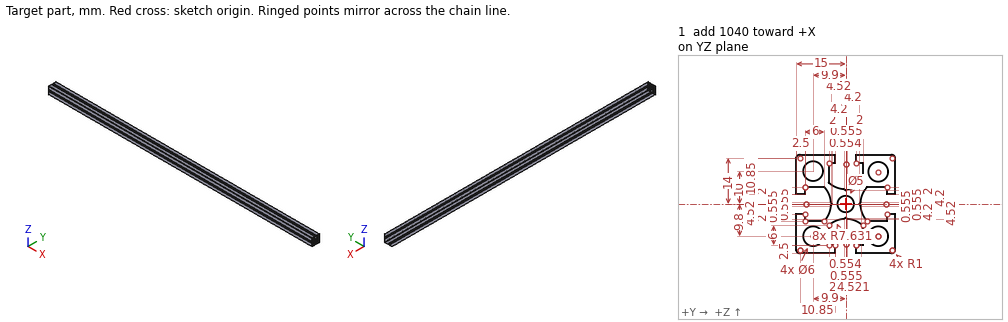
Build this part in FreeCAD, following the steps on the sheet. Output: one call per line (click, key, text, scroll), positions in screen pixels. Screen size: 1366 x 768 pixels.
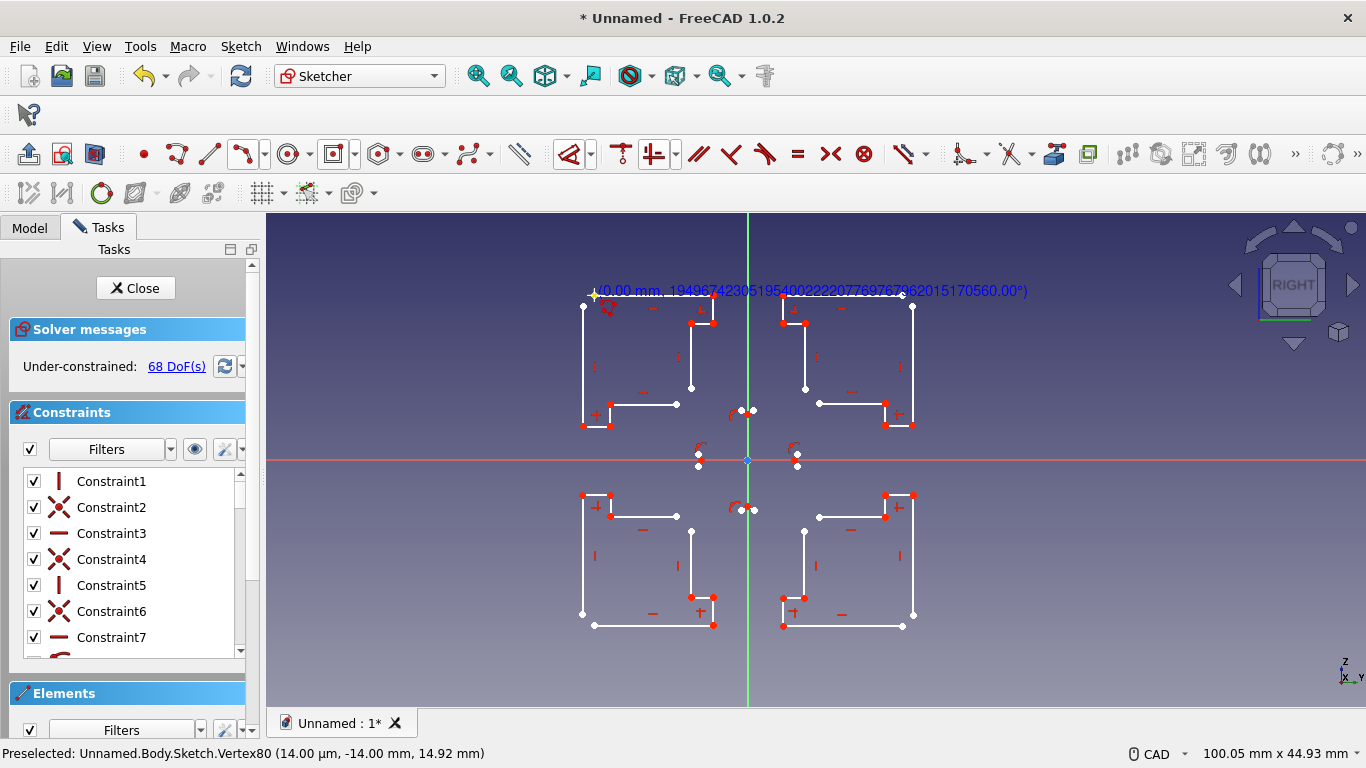
key(g)
key(3)
key(a)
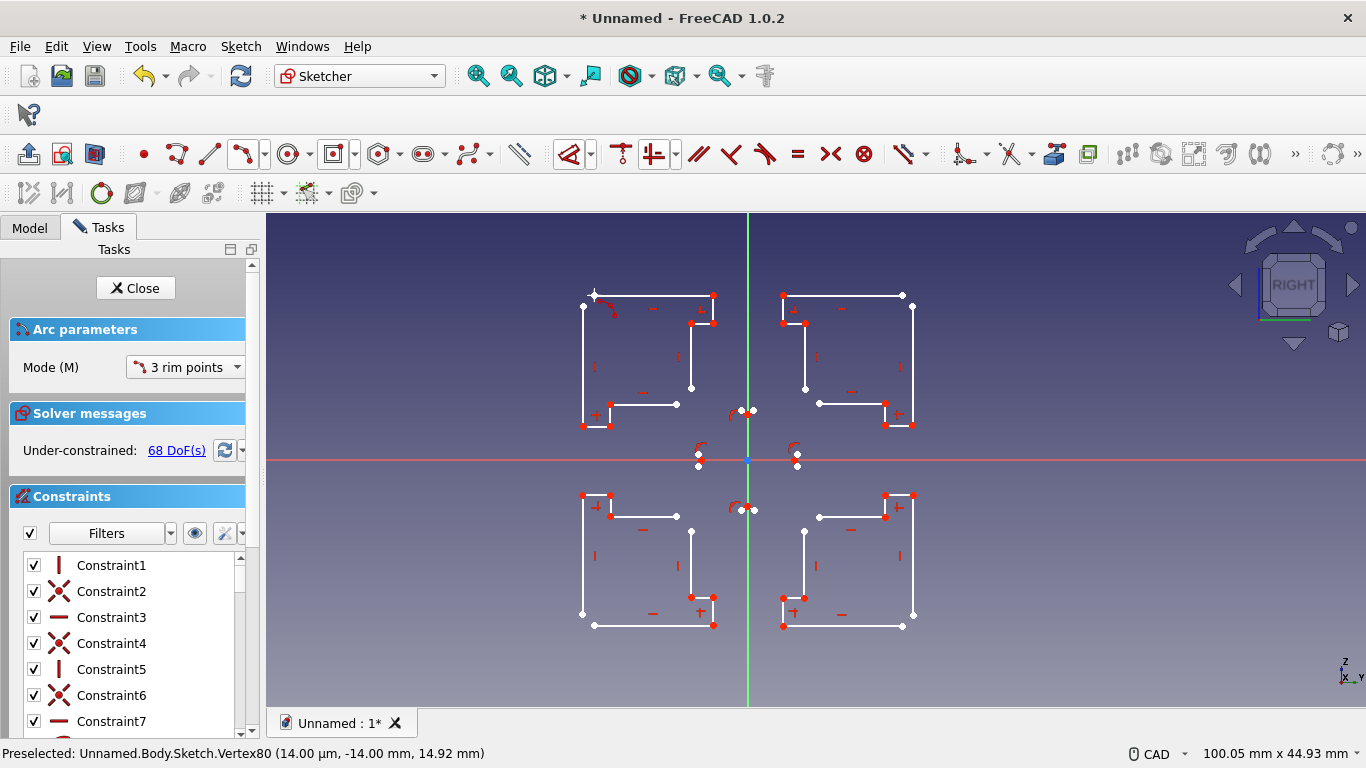
click(676, 405)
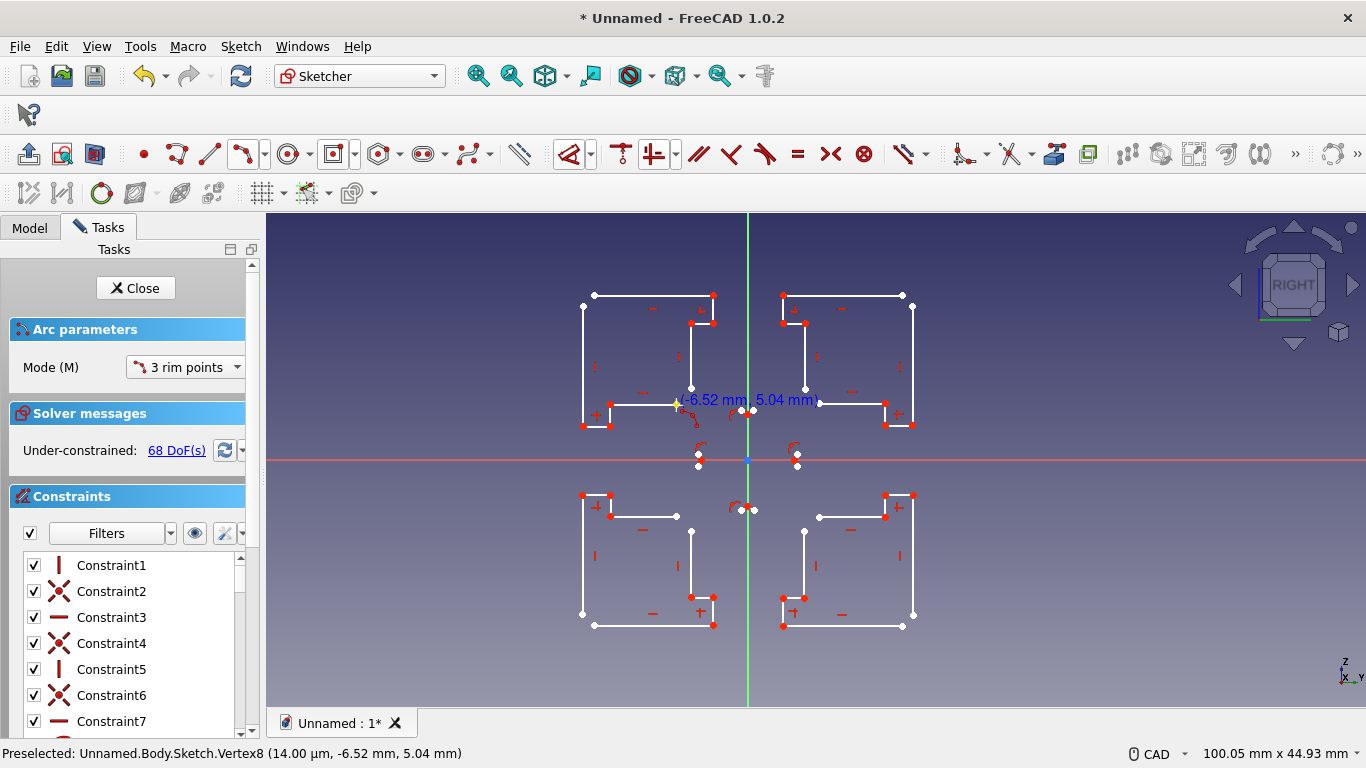
scroll(698, 454, up, 8)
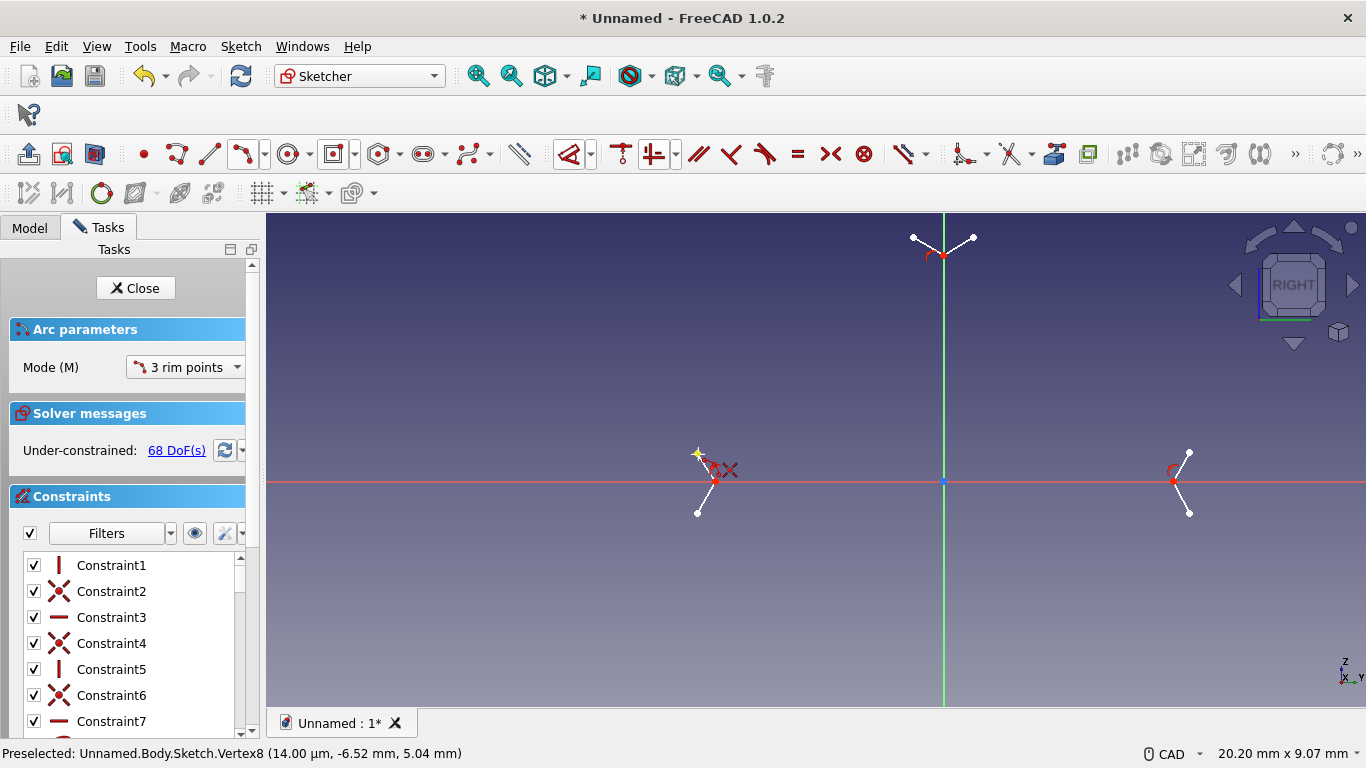
click(697, 454)
click(665, 317)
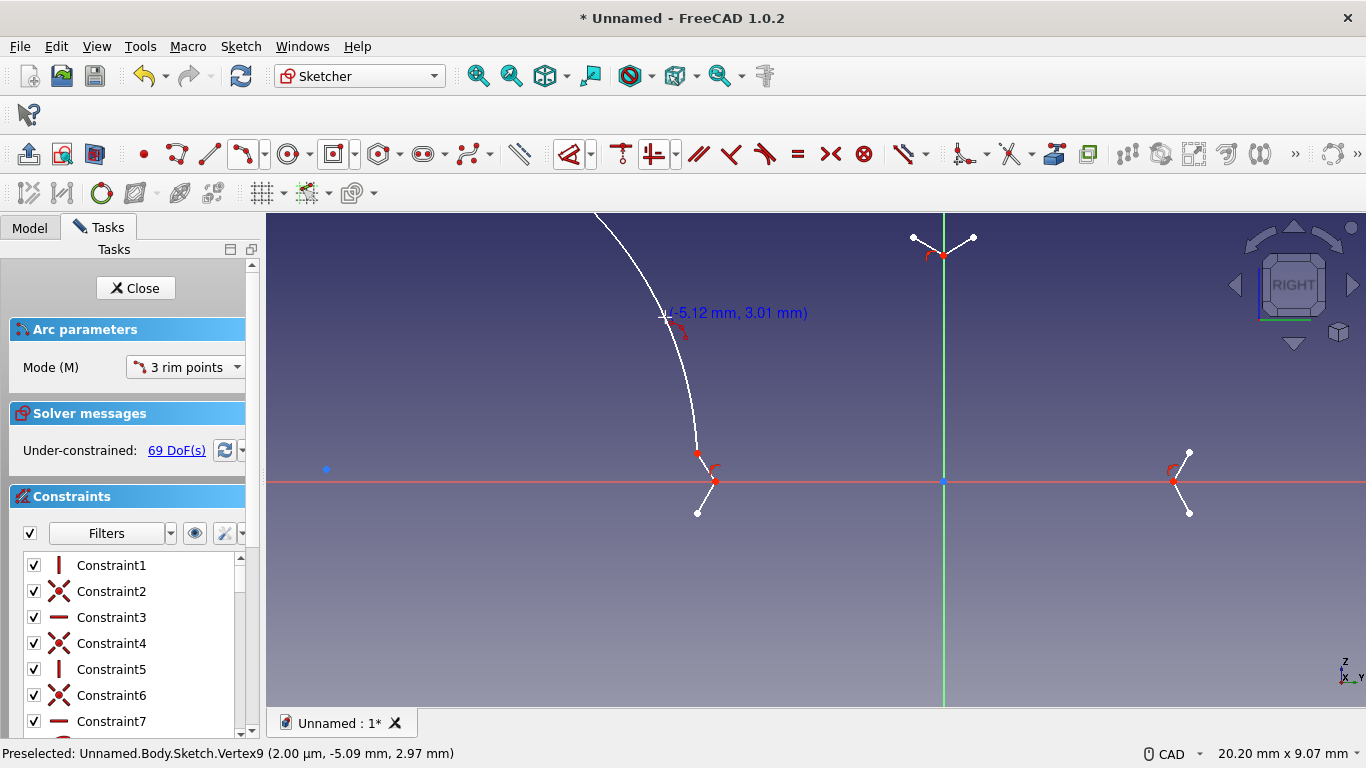
click(697, 514)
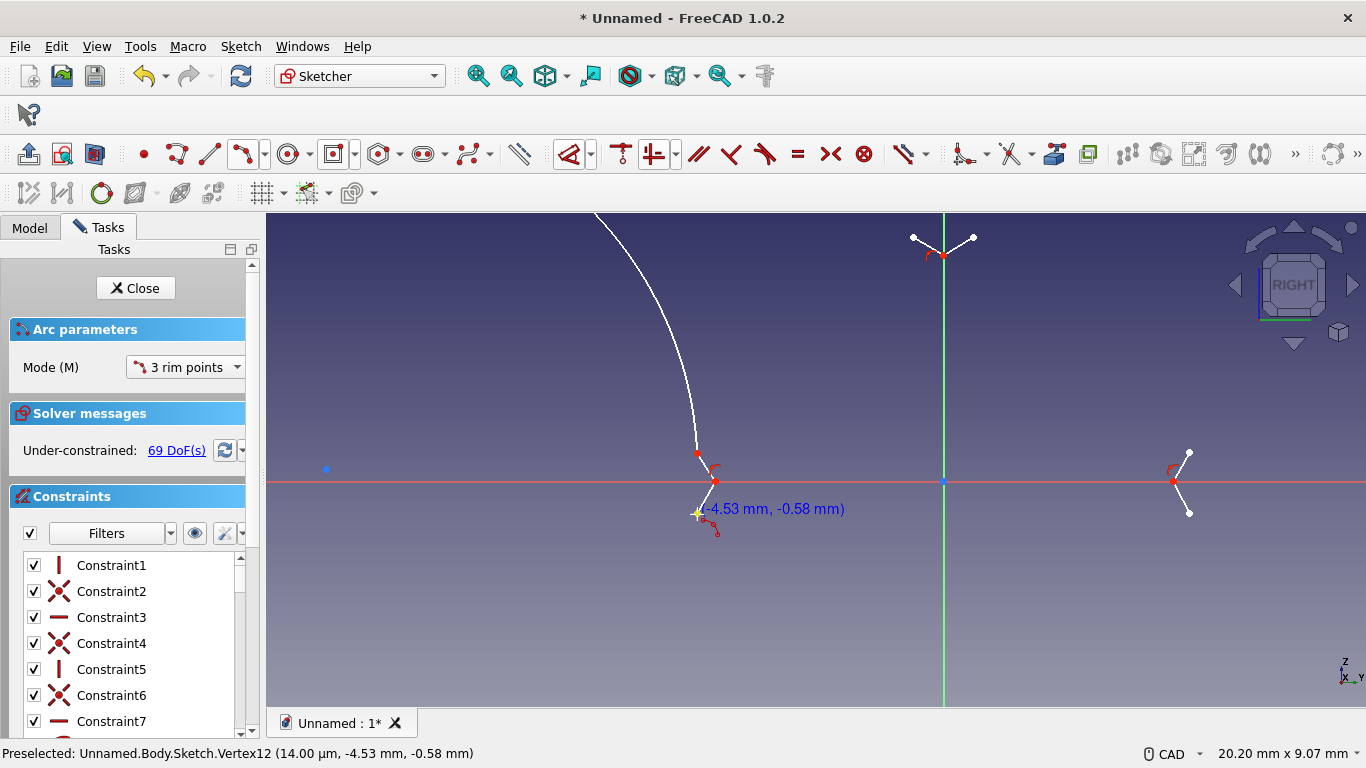
scroll(698, 454, down, 8)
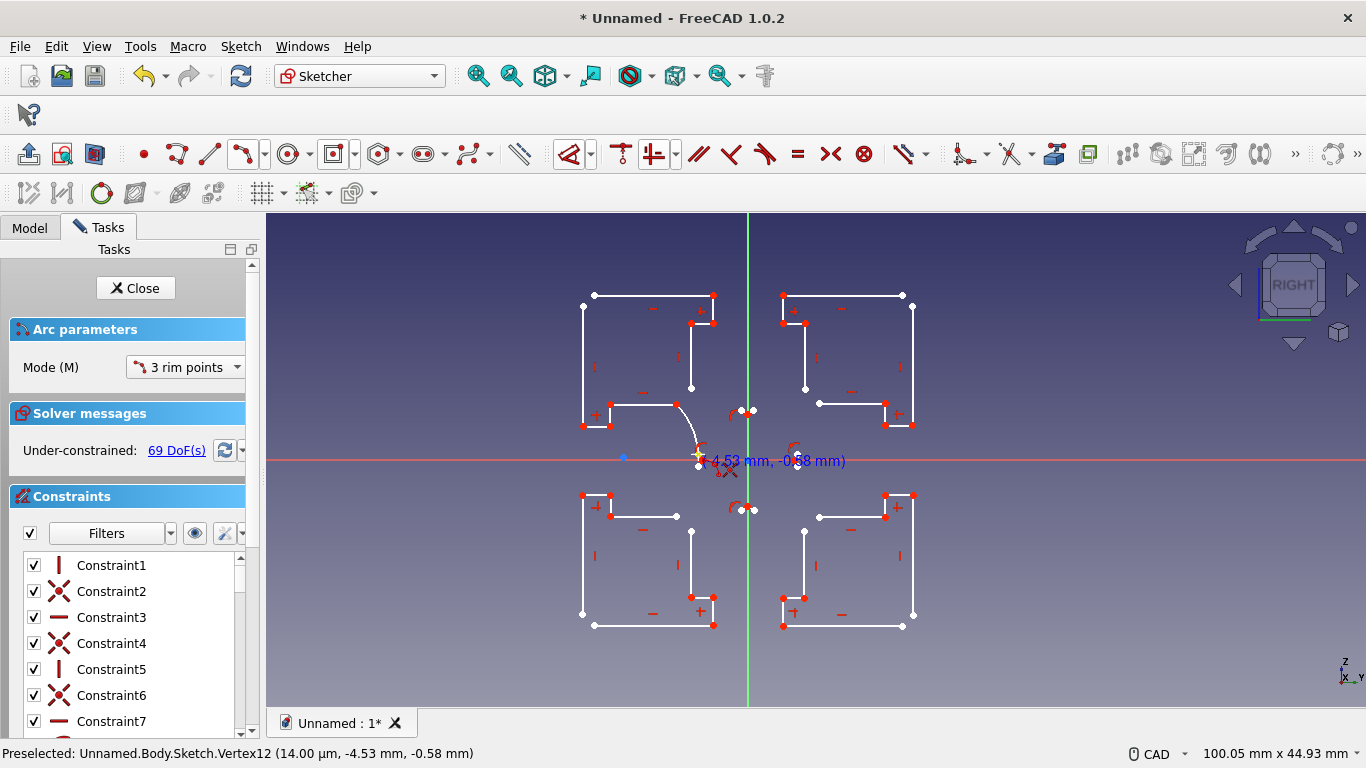
click(676, 517)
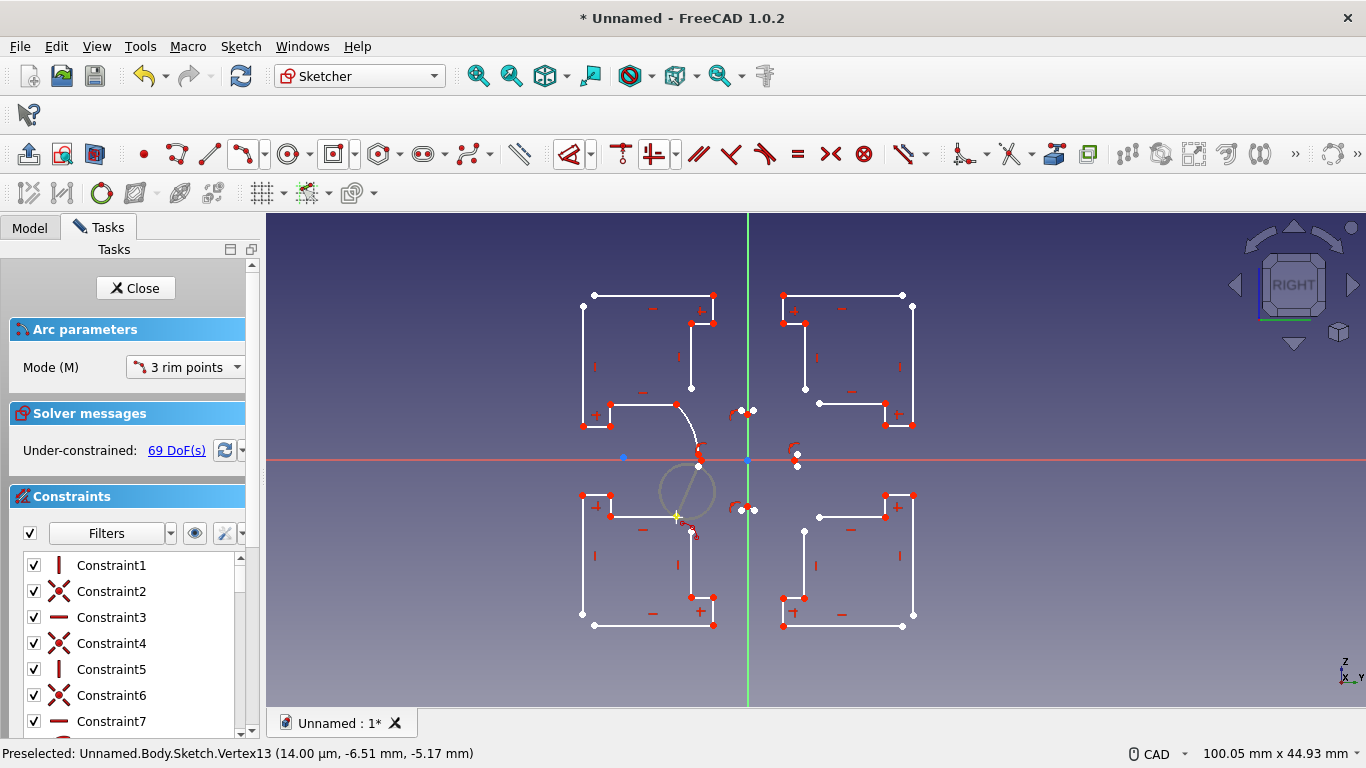
scroll(692, 493, up, 7)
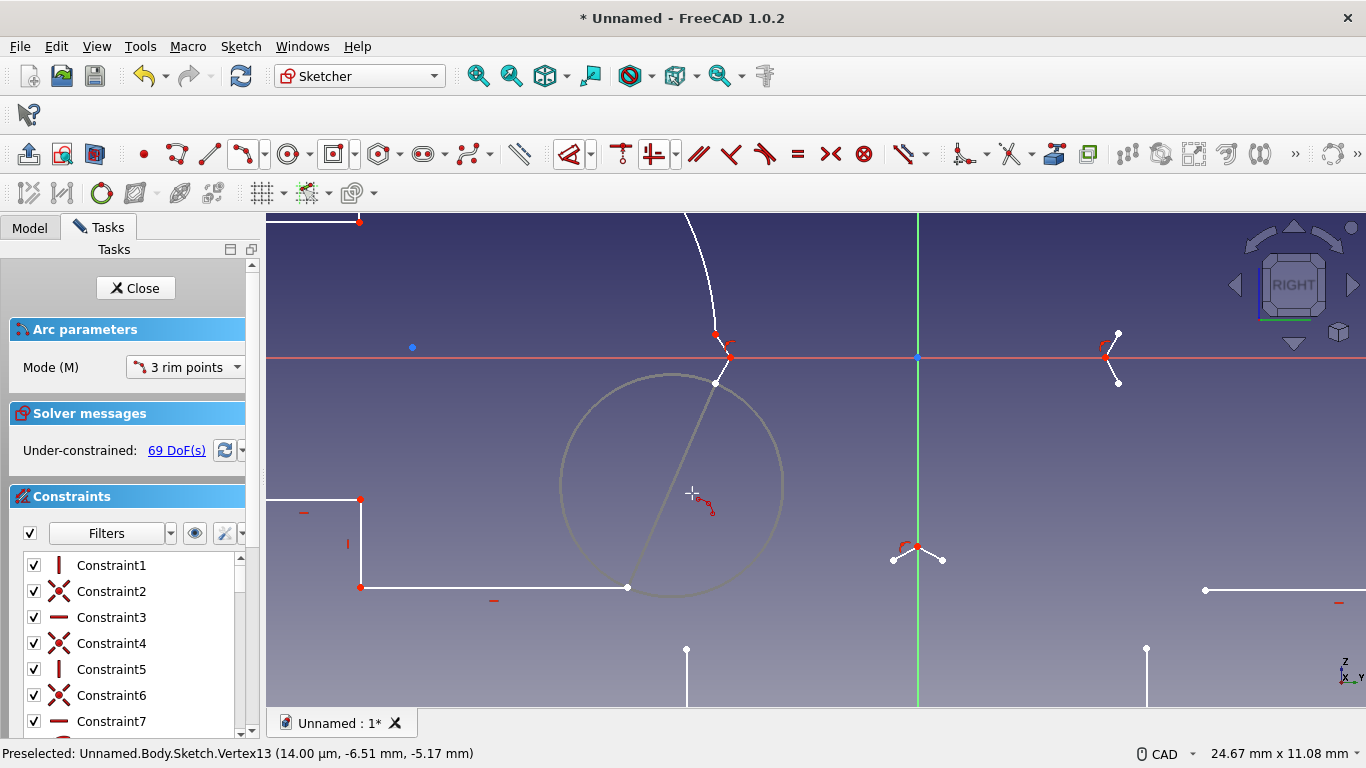
click(689, 492)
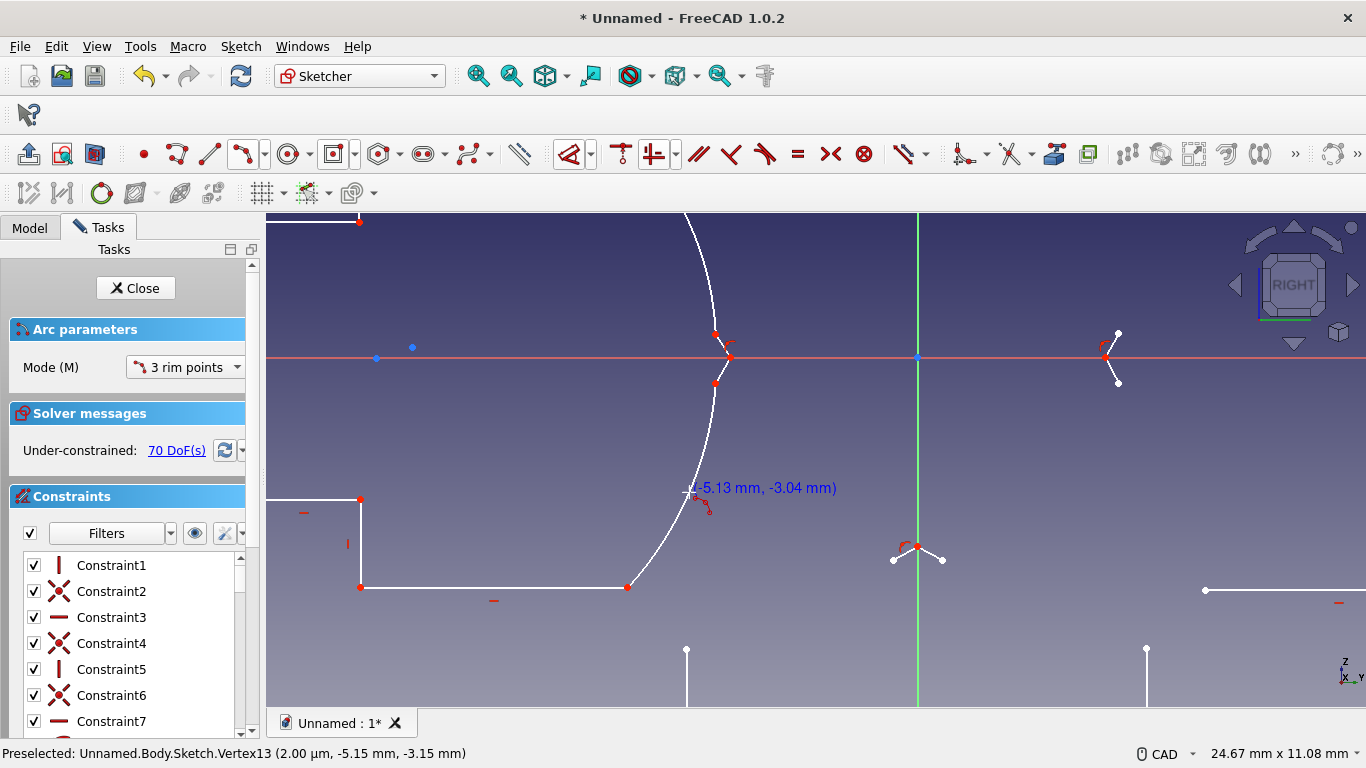
scroll(692, 494, down, 7)